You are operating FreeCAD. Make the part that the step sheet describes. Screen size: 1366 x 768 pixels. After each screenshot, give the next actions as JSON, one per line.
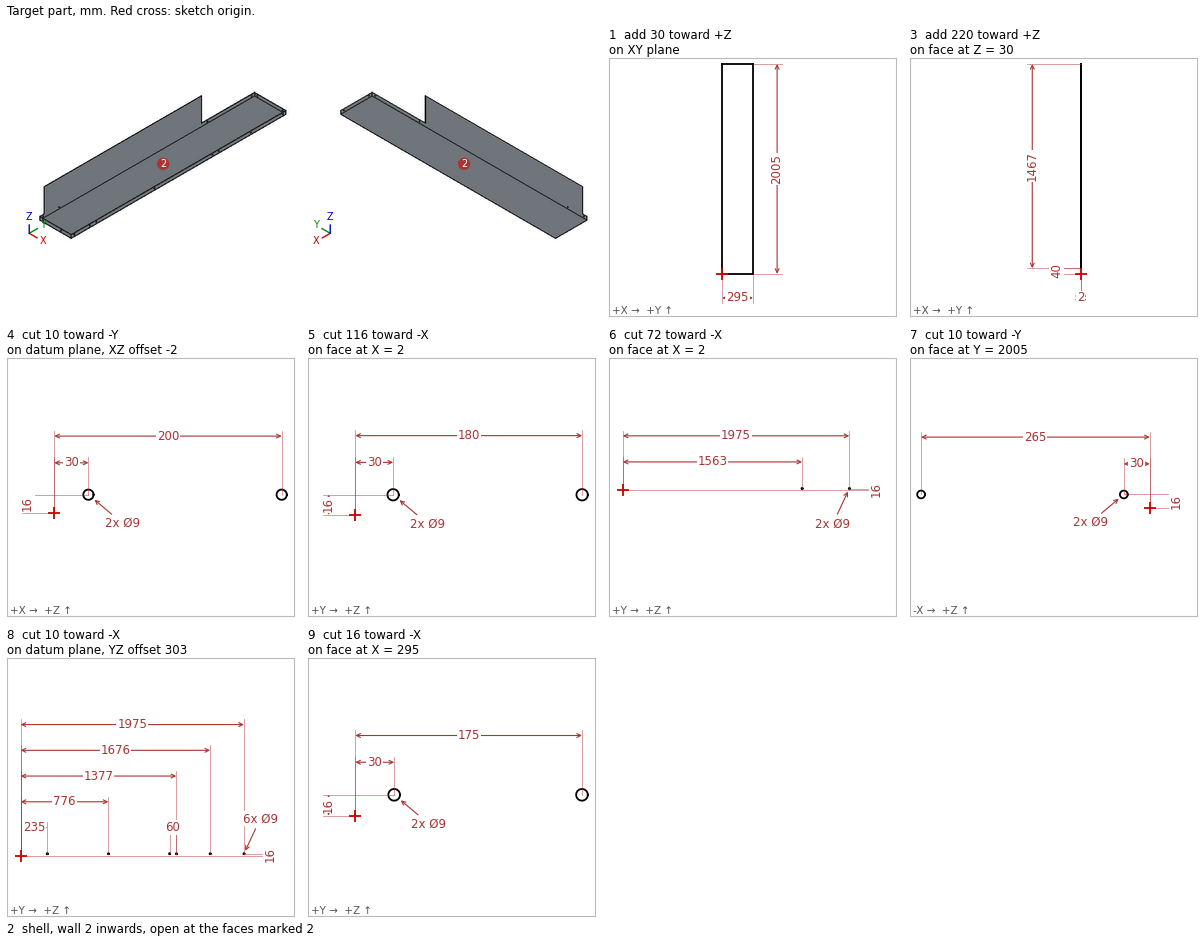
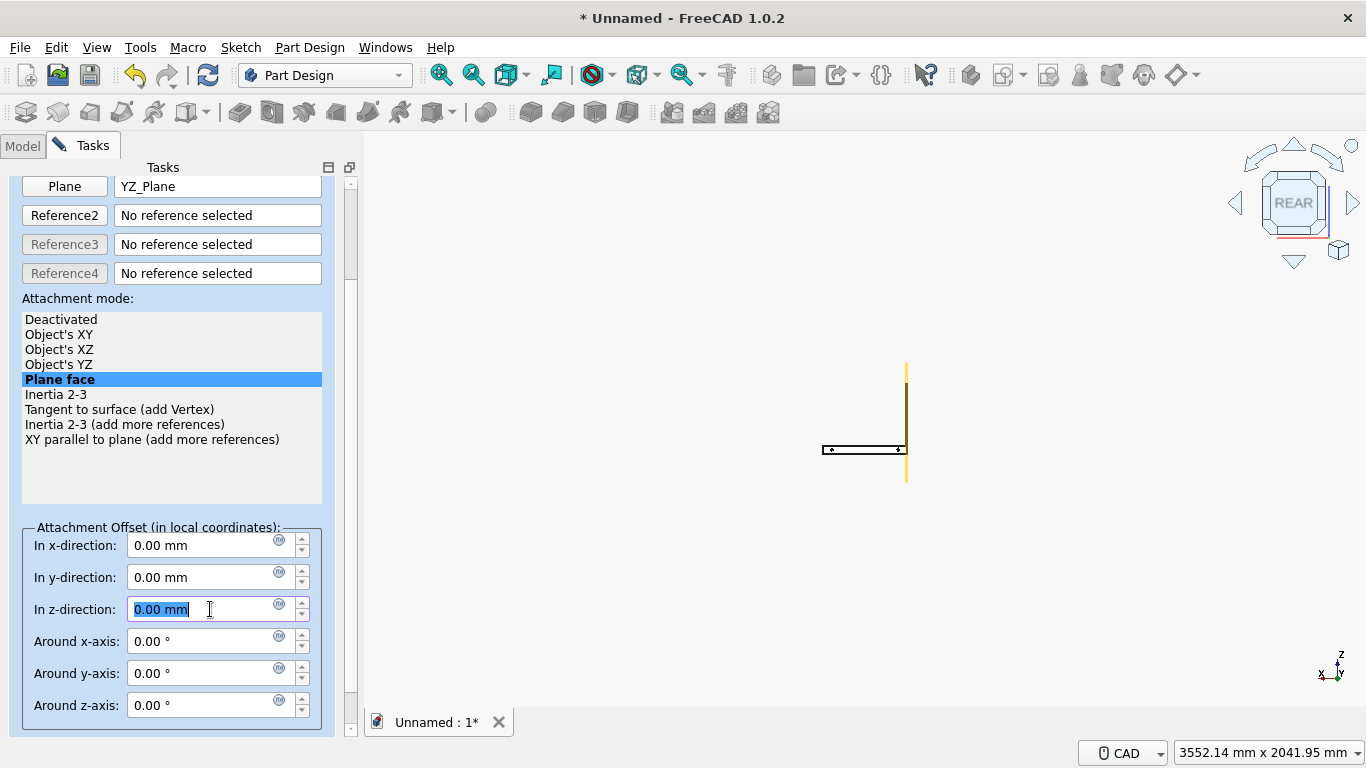
{"action": "type", "text": "303"}
{"action": "key", "text": "Tab"}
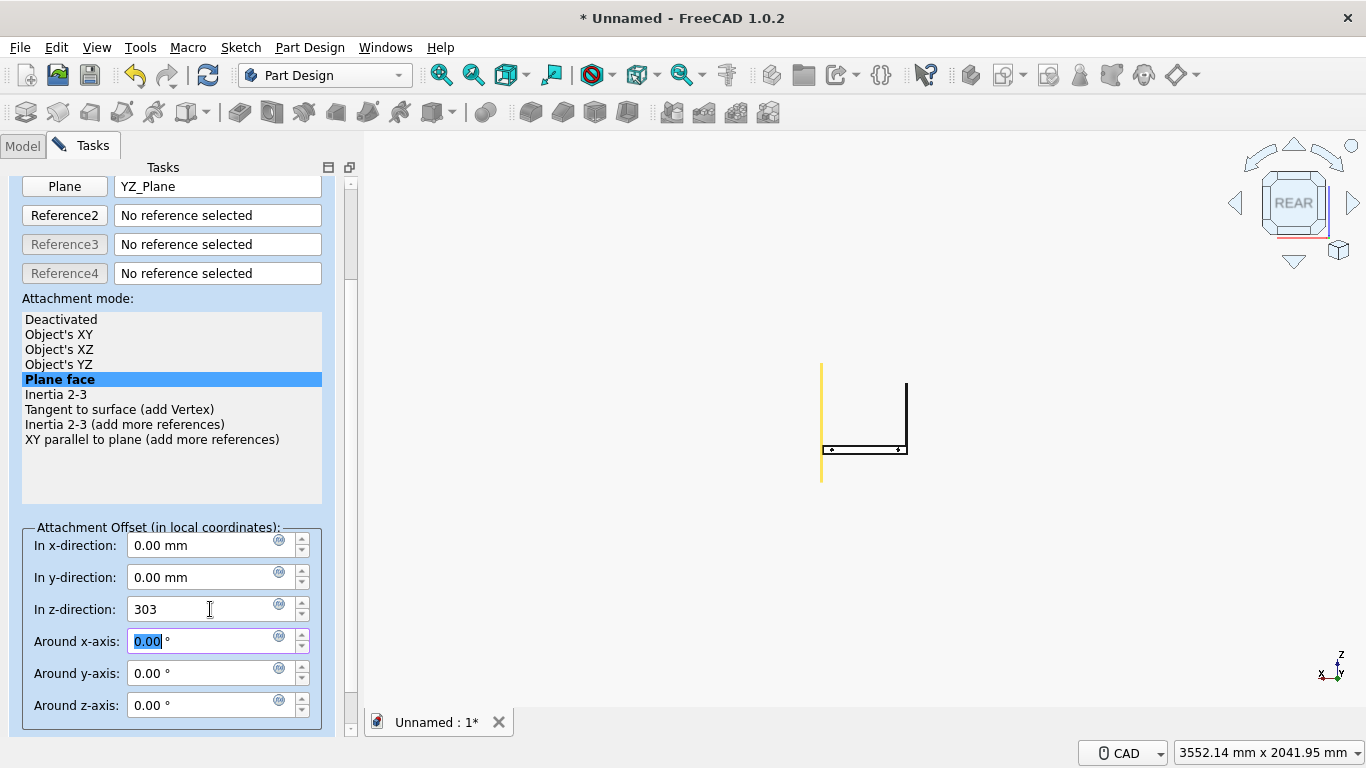
{"action": "scroll", "coordinate": [351, 456], "scroll_direction": "up", "scroll_amount": 3}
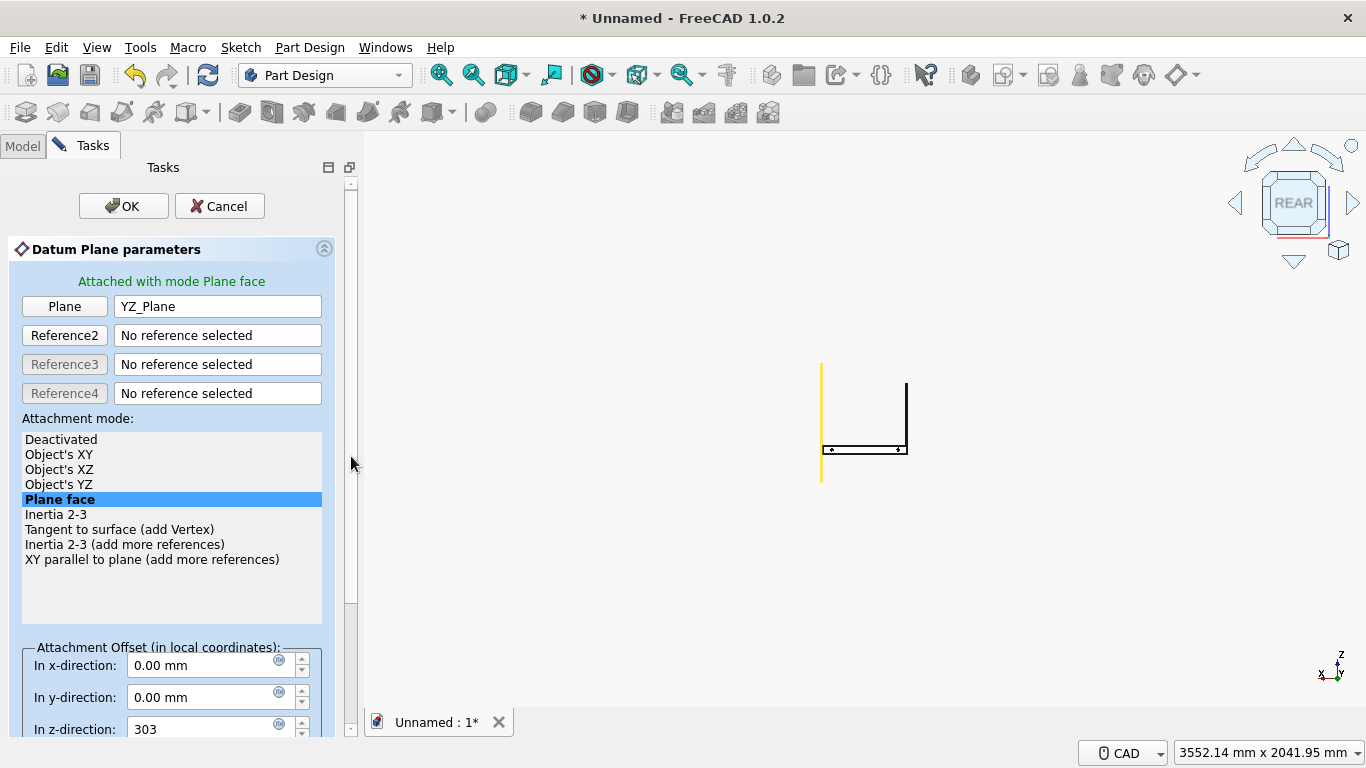
{"action": "left_click", "coordinate": [124, 206]}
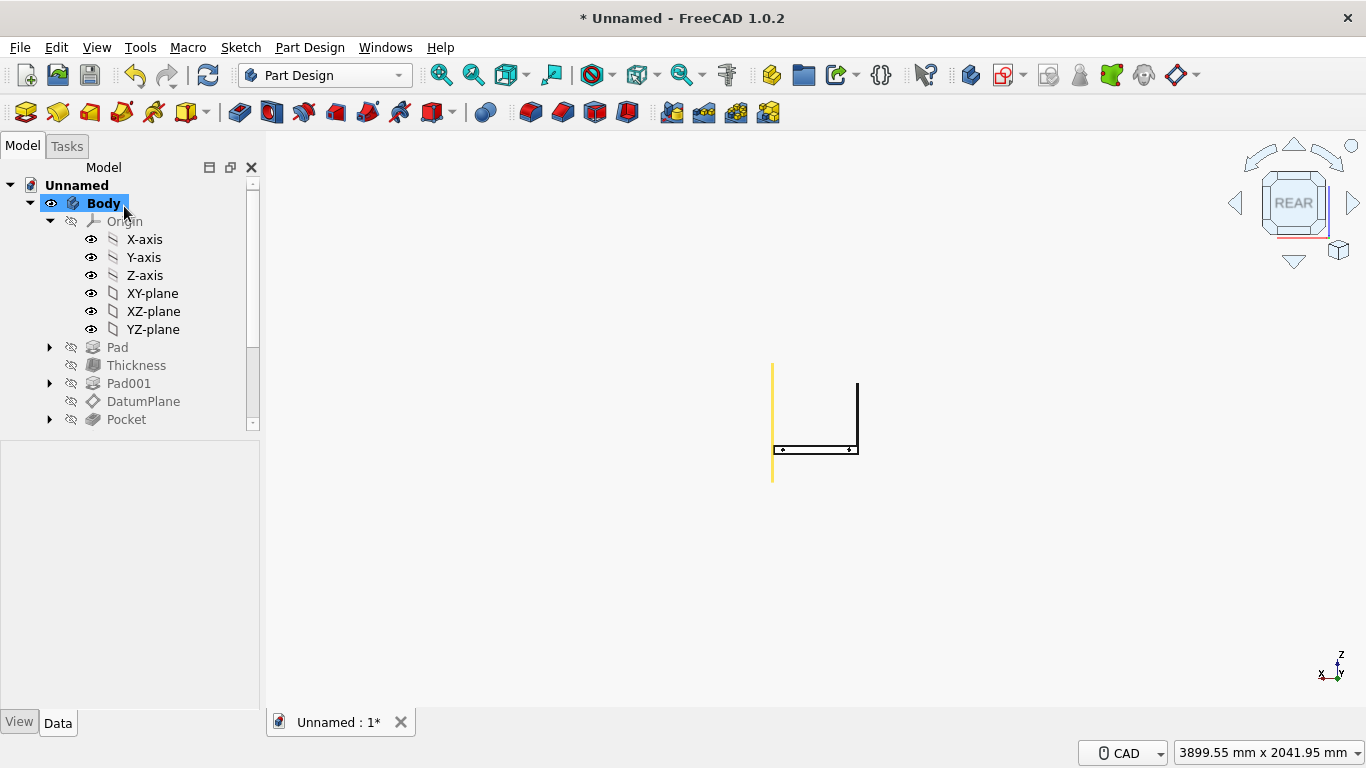
{"action": "scroll", "coordinate": [100, 307], "scroll_direction": "down", "scroll_amount": 3}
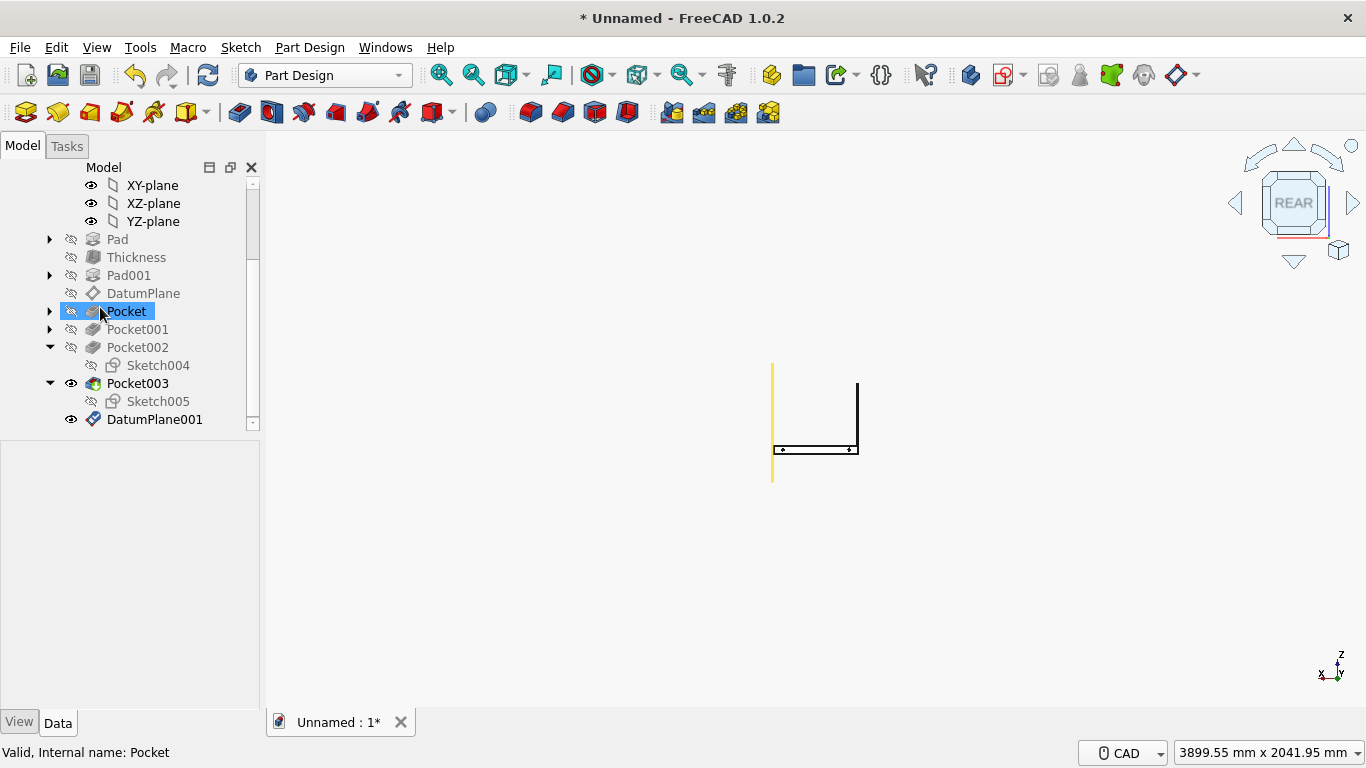
{"action": "left_click", "coordinate": [116, 419]}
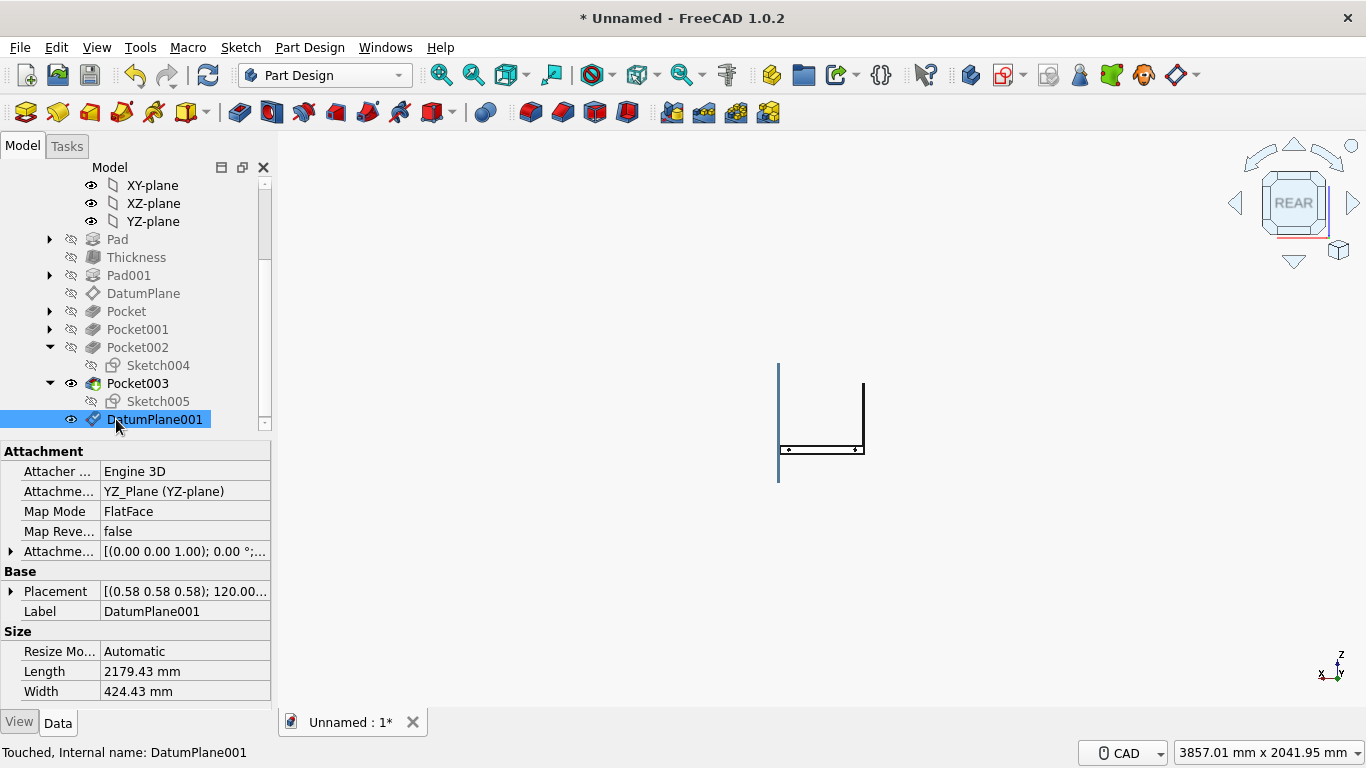
{"action": "left_click", "coordinate": [1004, 76]}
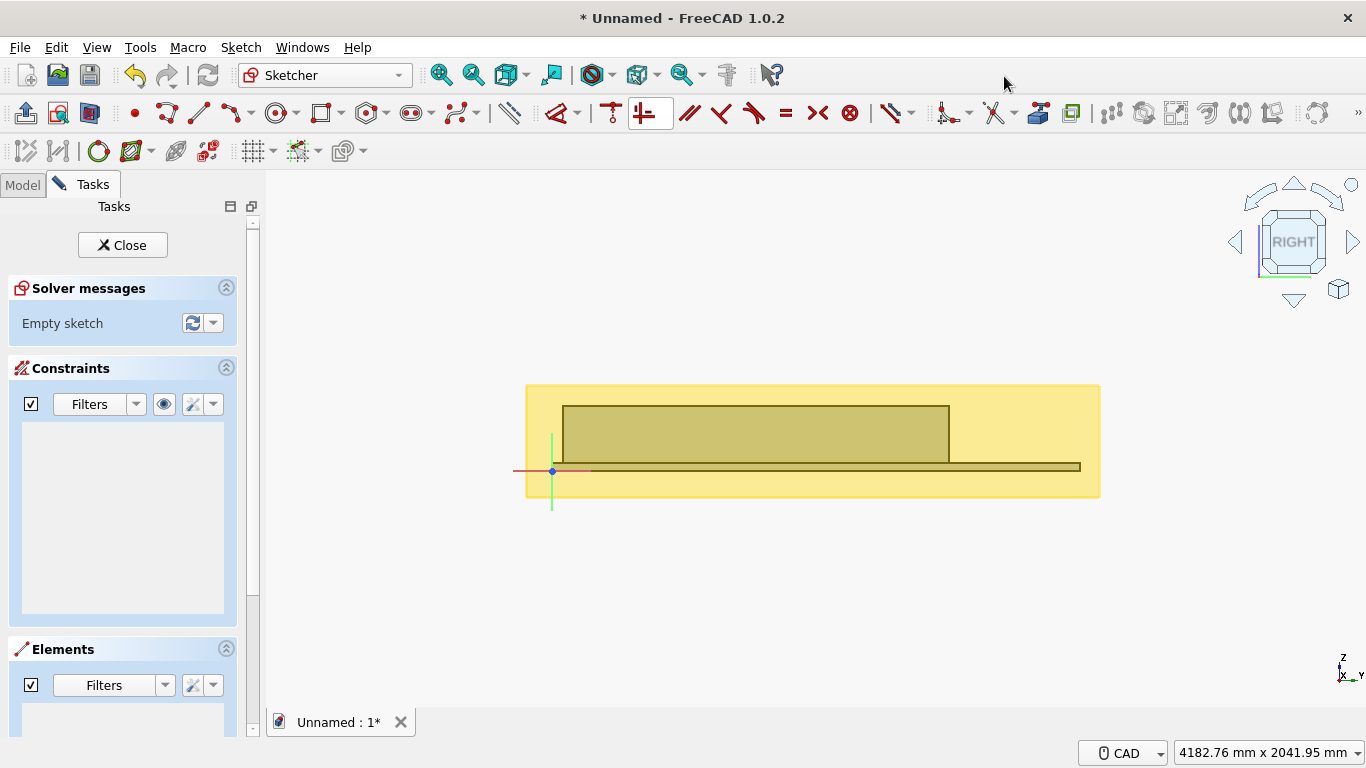
{"action": "left_click", "coordinate": [276, 114]}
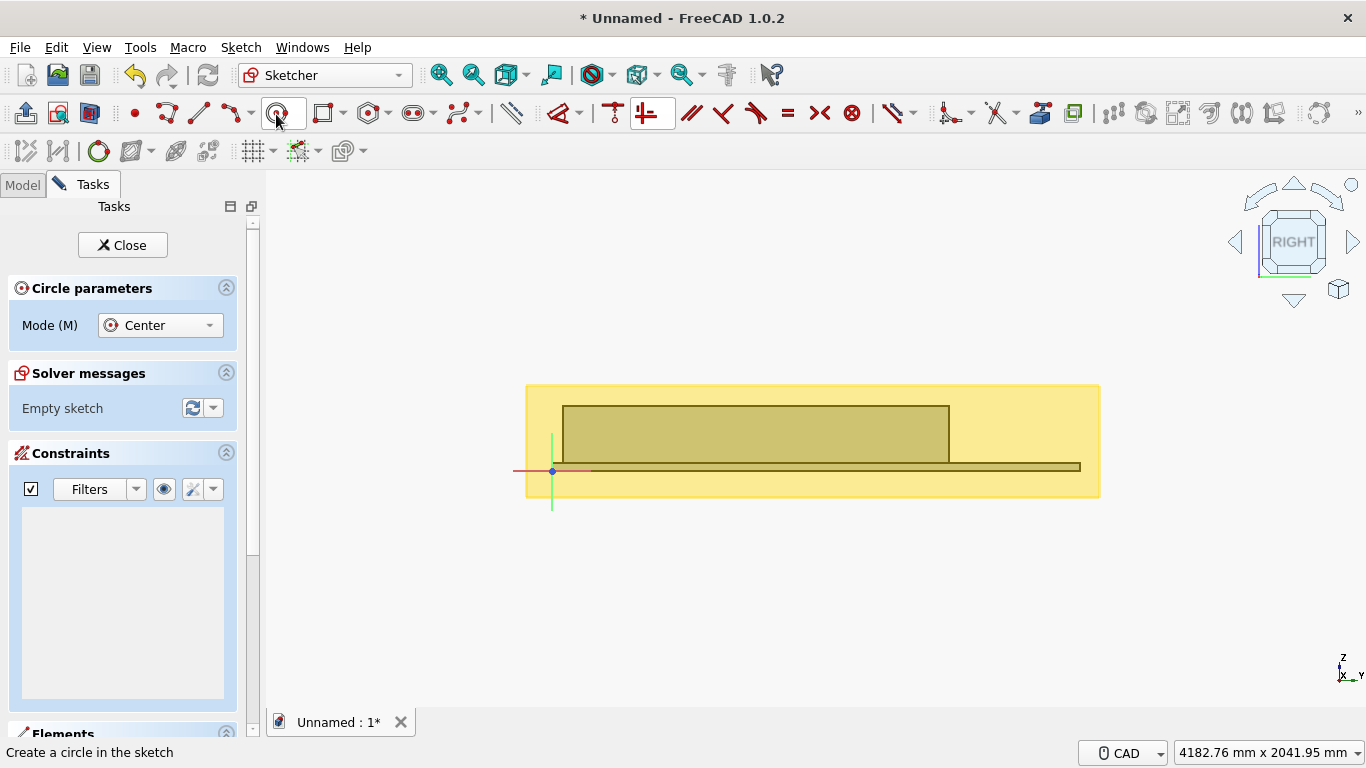
{"action": "scroll", "coordinate": [1072, 467], "scroll_direction": "up", "scroll_amount": 15}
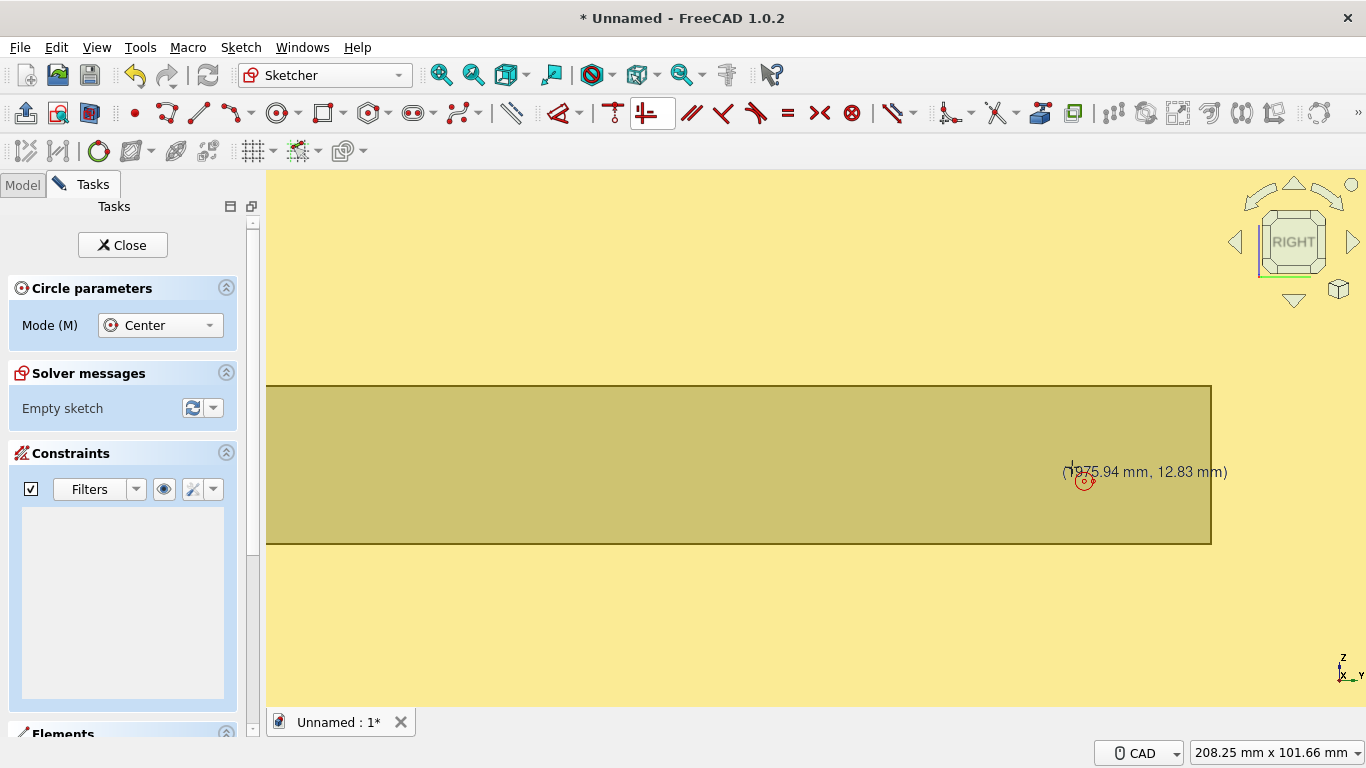
{"action": "scroll", "coordinate": [1065, 435], "scroll_direction": "down", "scroll_amount": 14}